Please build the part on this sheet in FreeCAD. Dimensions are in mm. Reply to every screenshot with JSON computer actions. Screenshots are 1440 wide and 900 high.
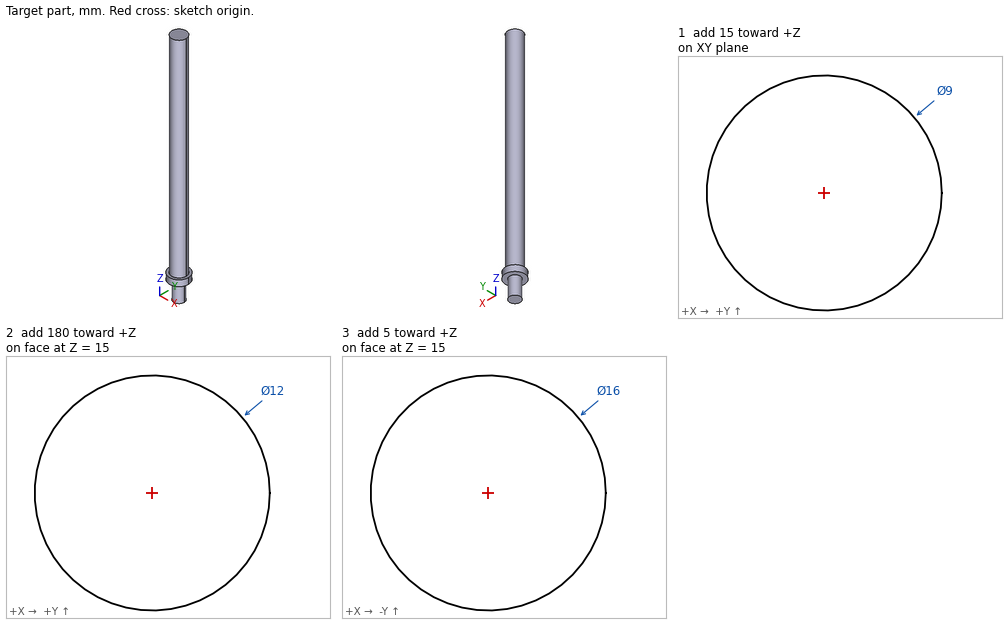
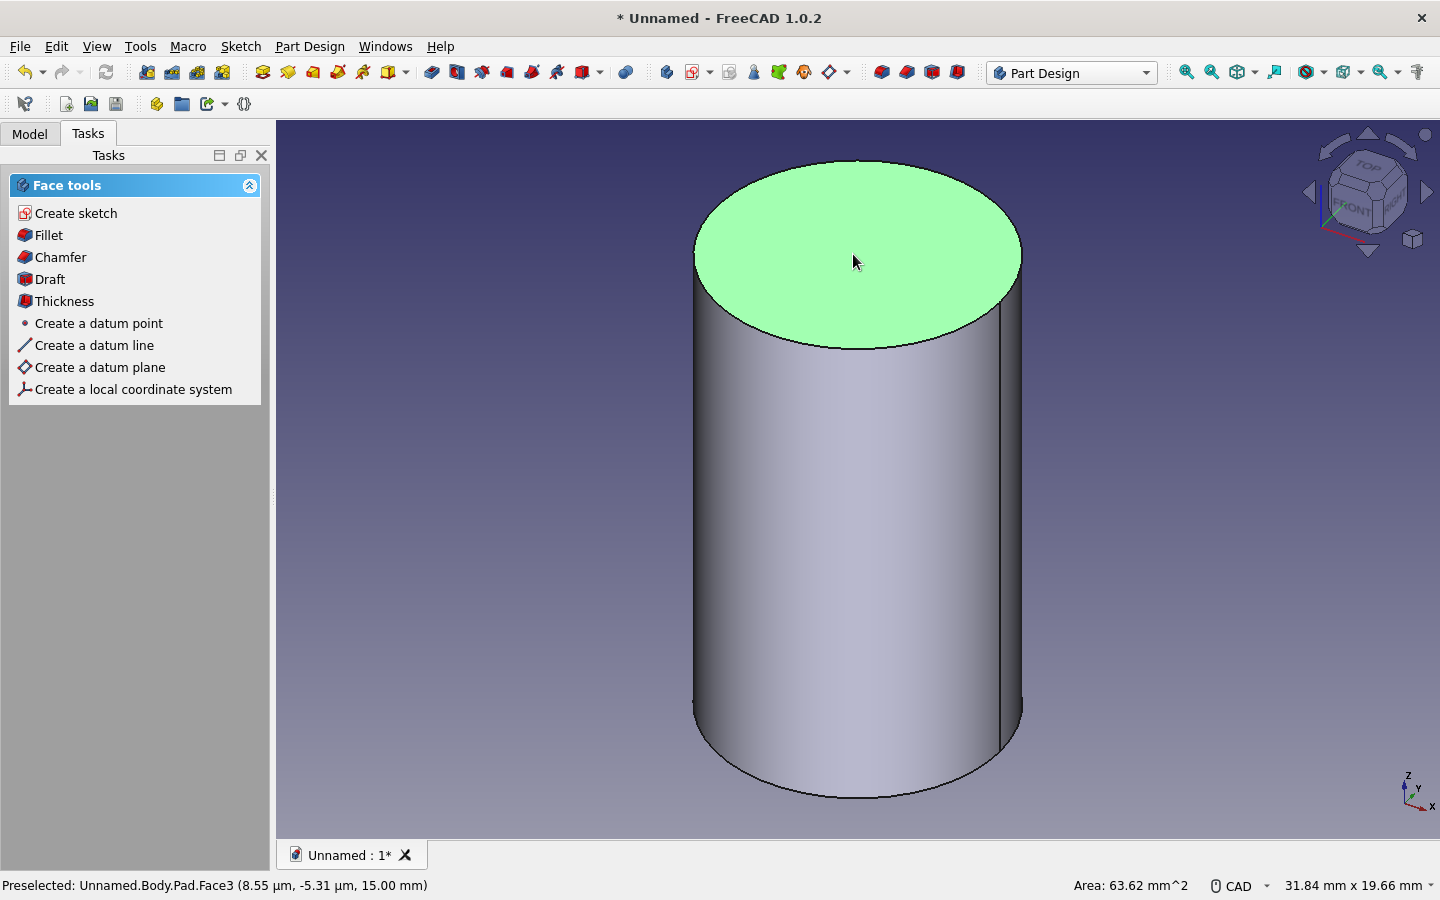
{"action": "left_click", "coordinate": [692, 72]}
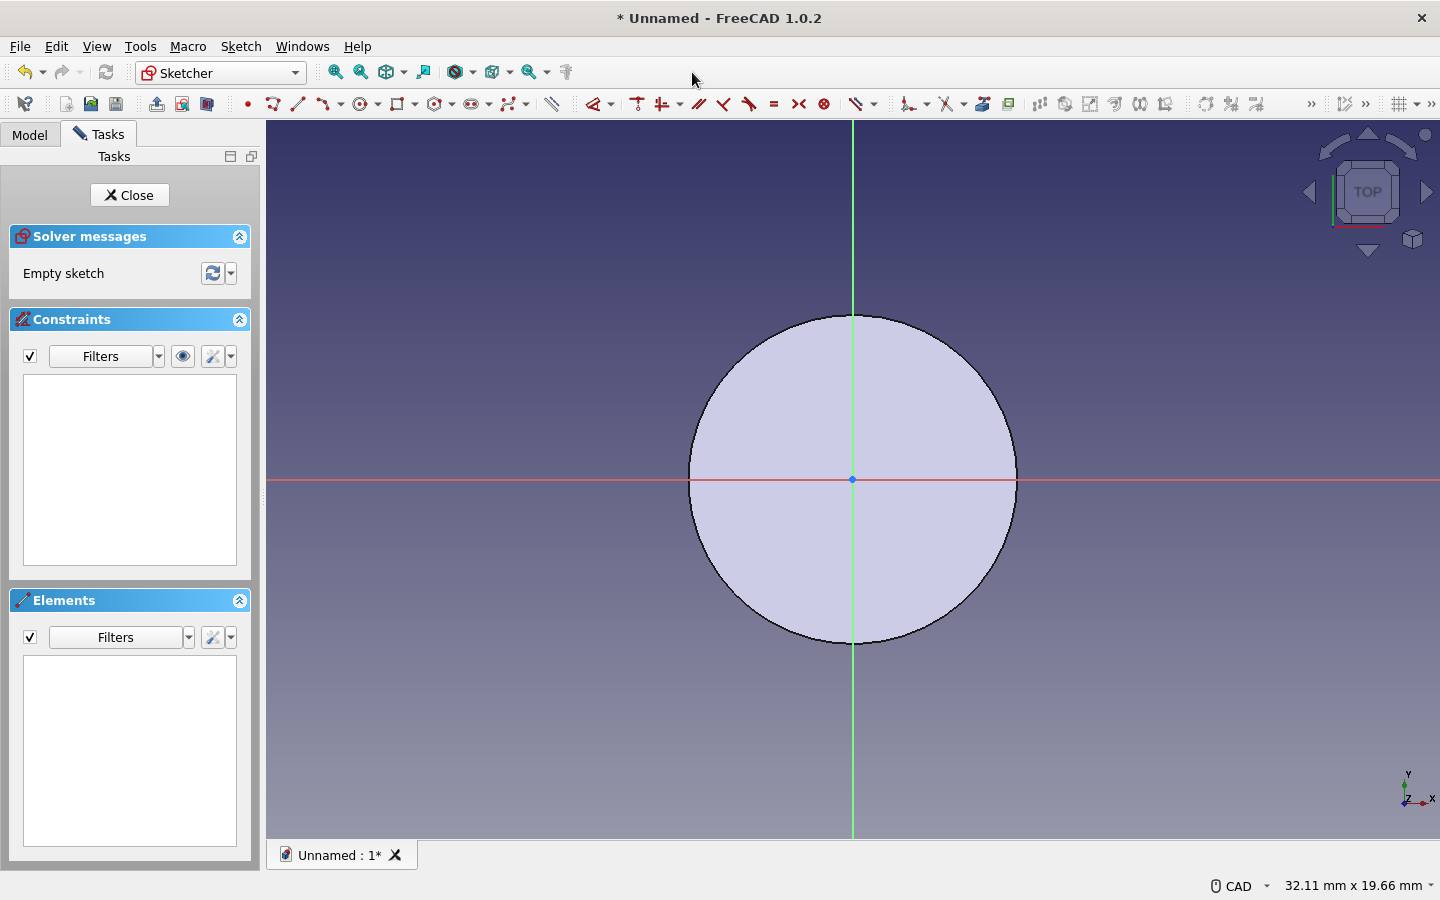
{"action": "key", "text": "g c"}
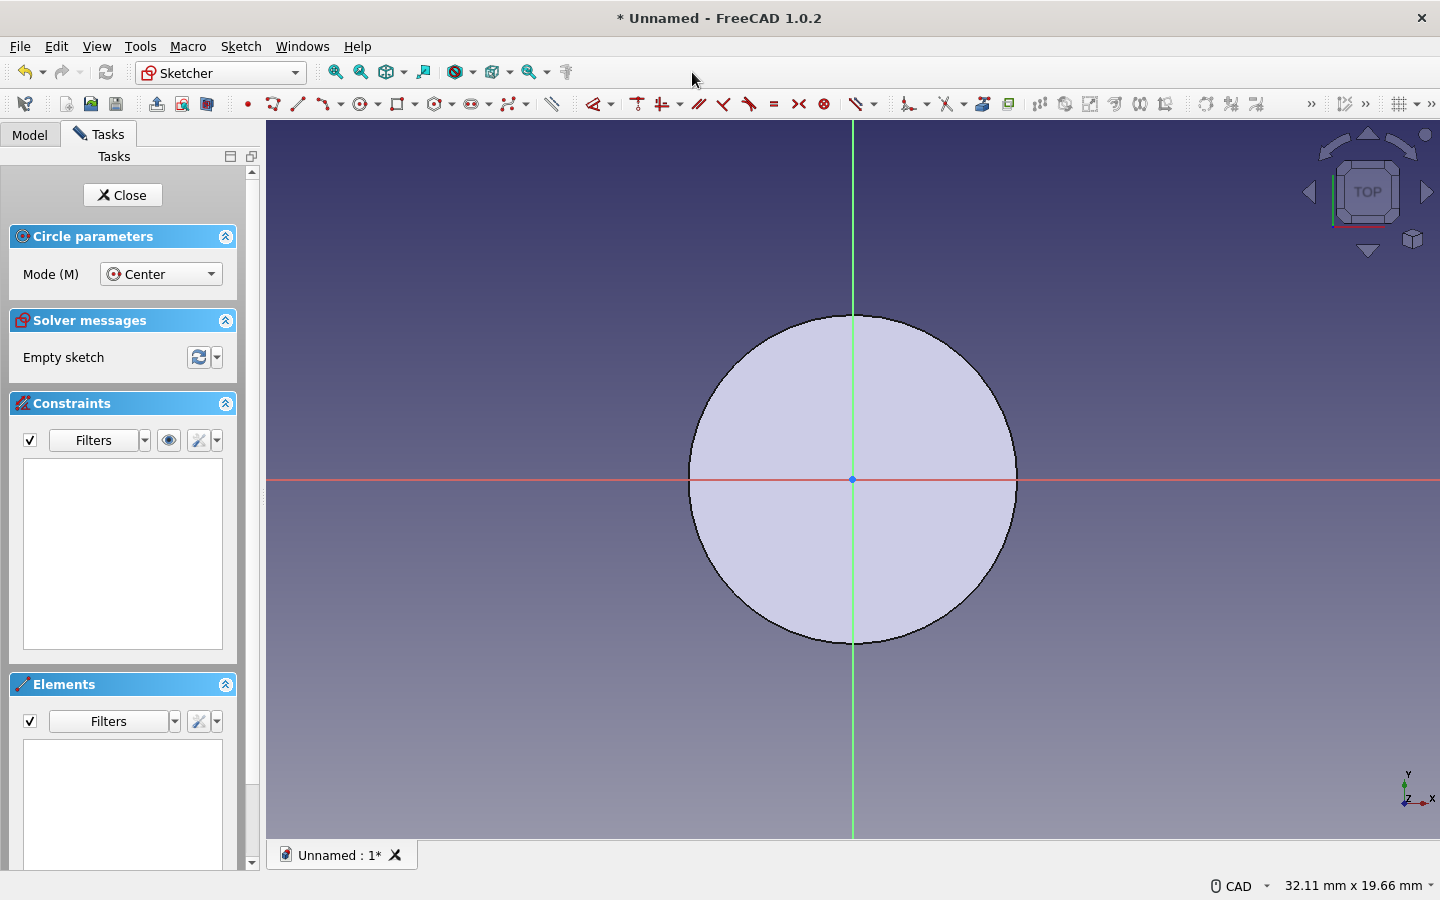
{"action": "left_click", "coordinate": [853, 480]}
{"action": "left_click", "coordinate": [1008, 324]}
{"action": "key", "text": "Escape"}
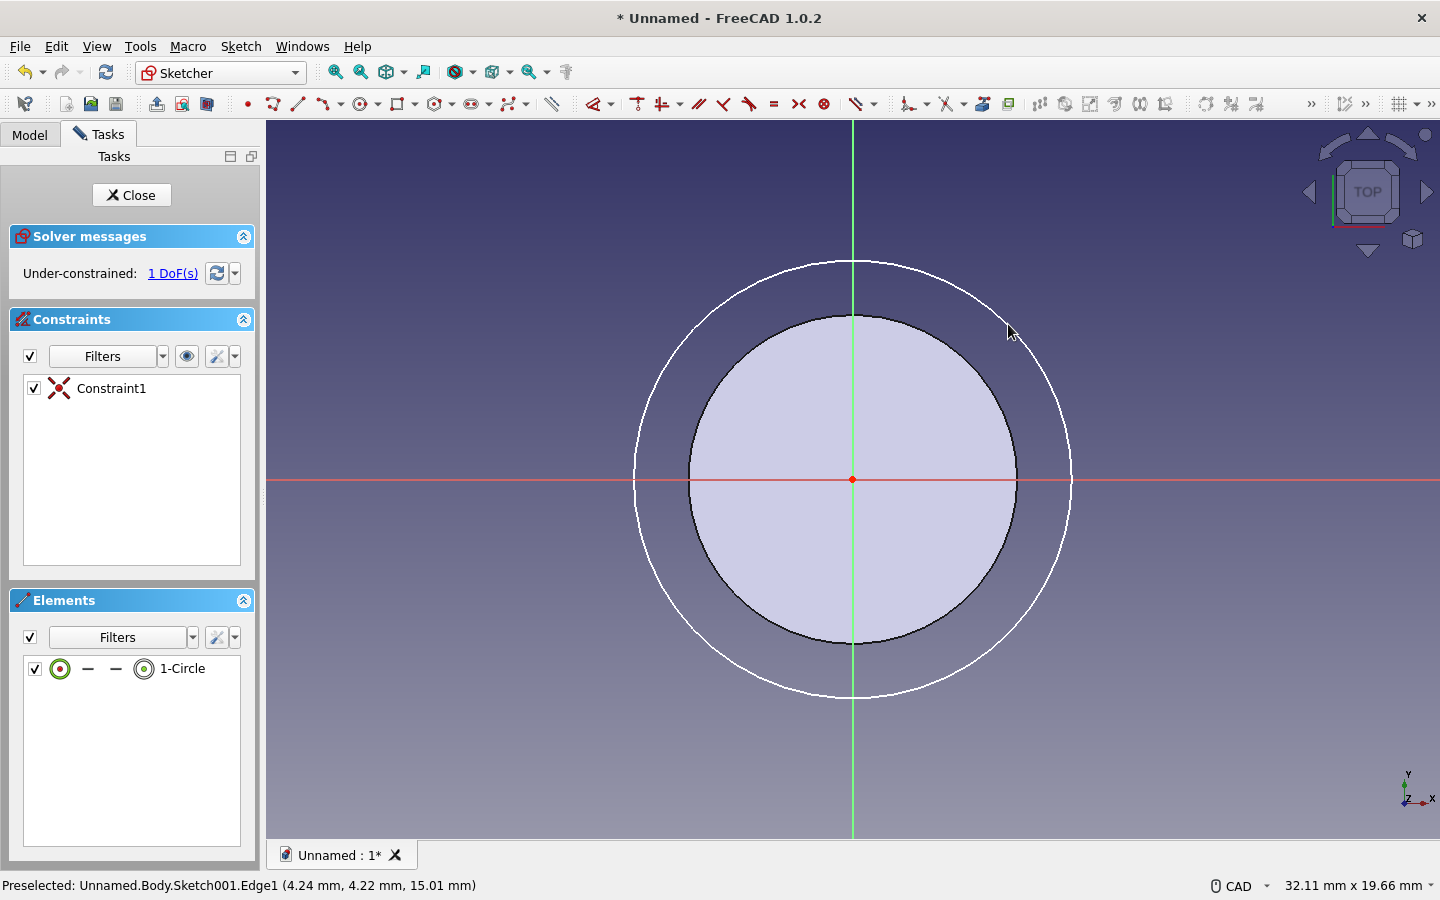
{"action": "left_click", "coordinate": [592, 104]}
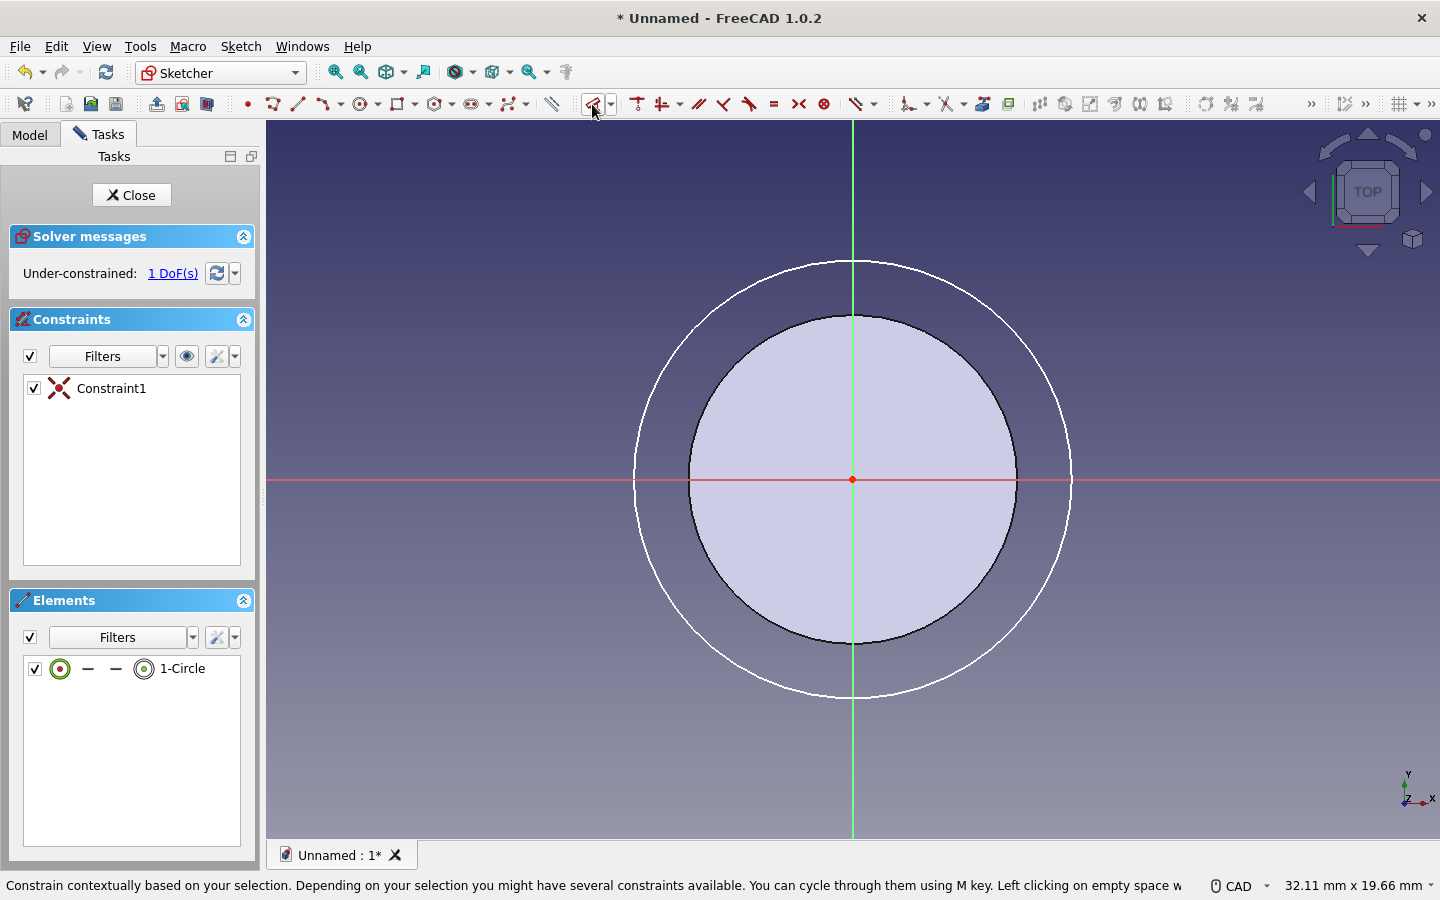
{"action": "left_click", "coordinate": [1007, 324]}
{"action": "left_click", "coordinate": [1030, 301]}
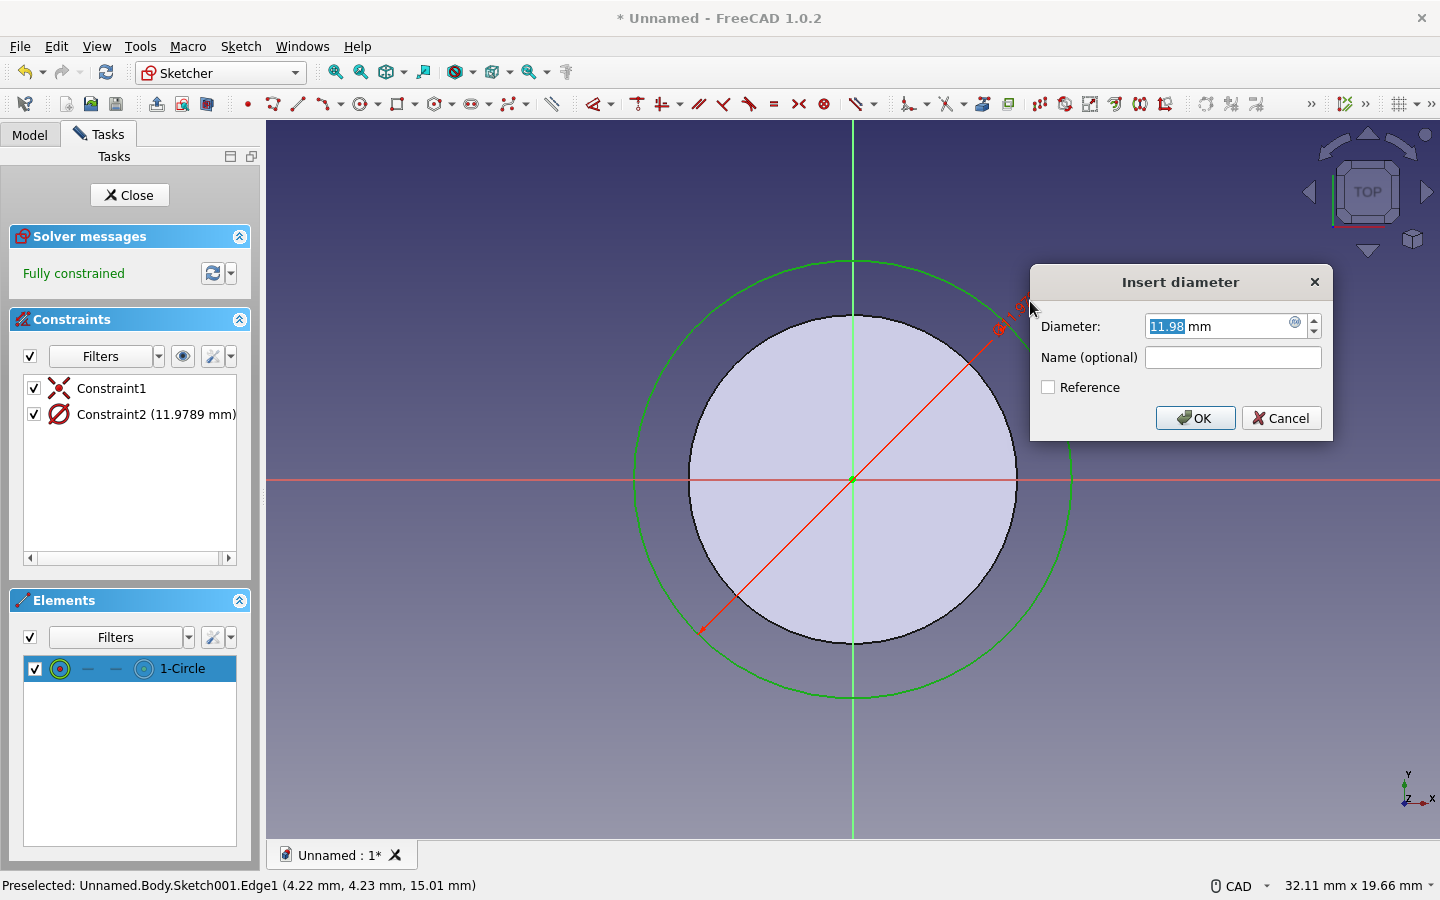
{"action": "type", "text": "12"}
{"action": "key", "text": "Return"}
{"action": "key", "text": "Escape"}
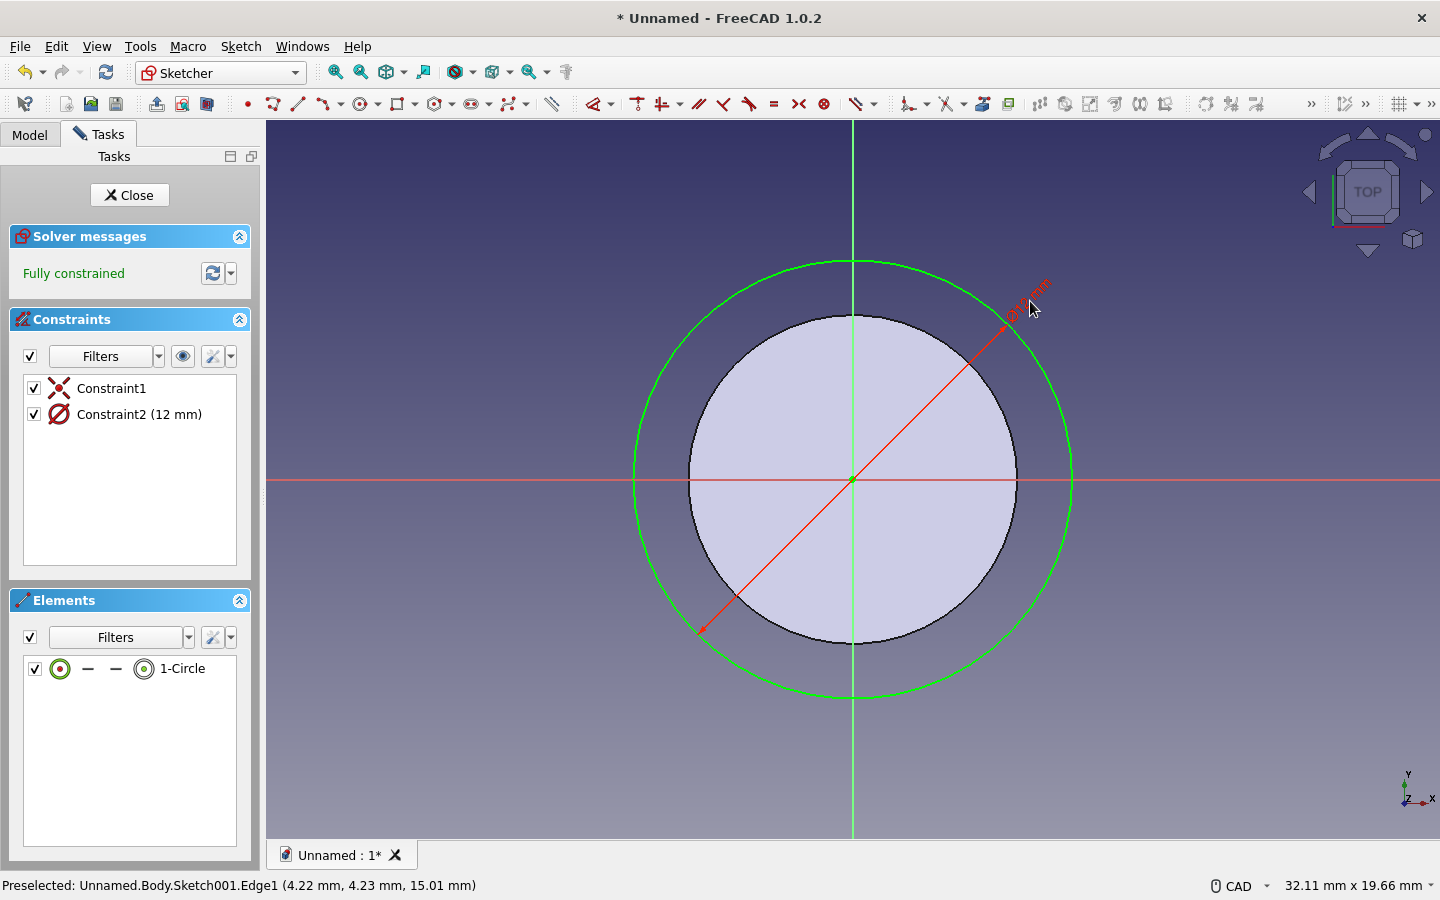
{"action": "left_click", "coordinate": [130, 195]}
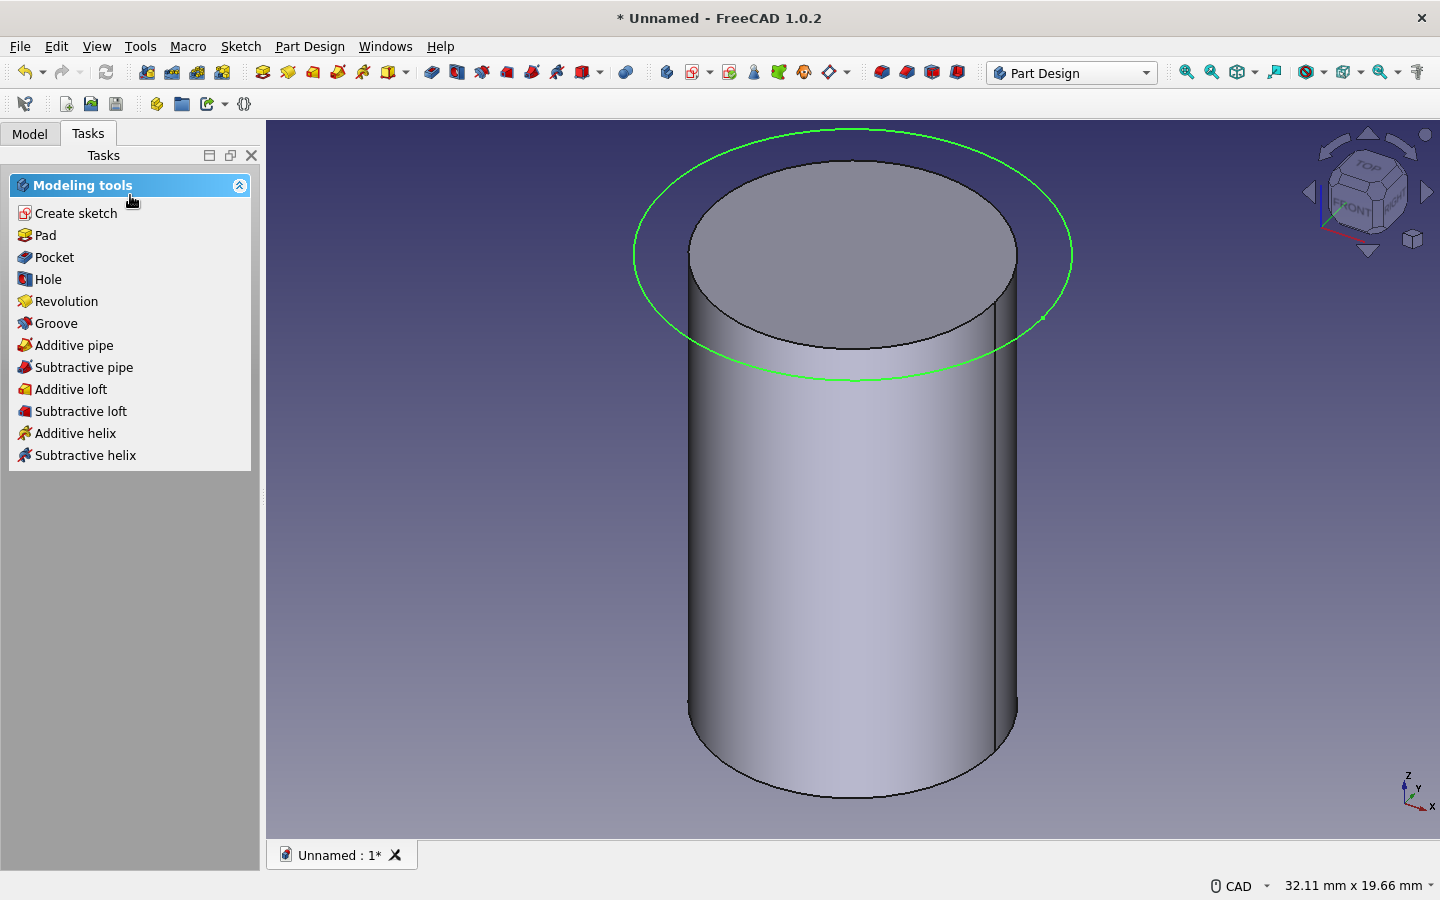
{"action": "left_click", "coordinate": [263, 72]}